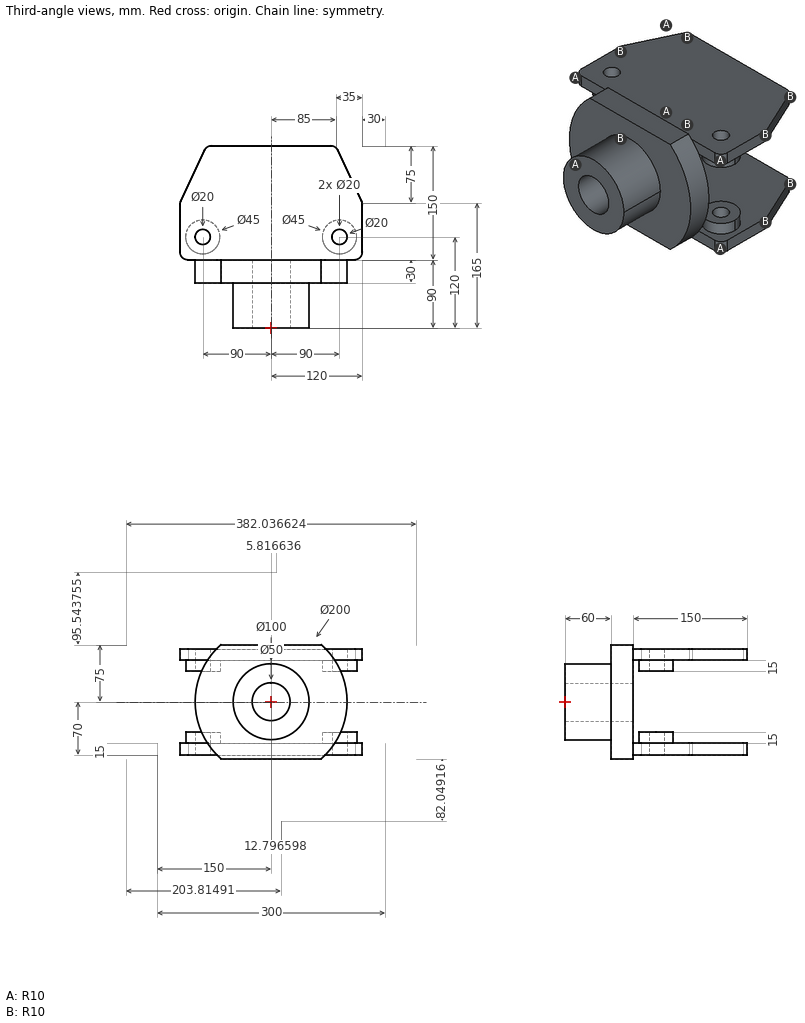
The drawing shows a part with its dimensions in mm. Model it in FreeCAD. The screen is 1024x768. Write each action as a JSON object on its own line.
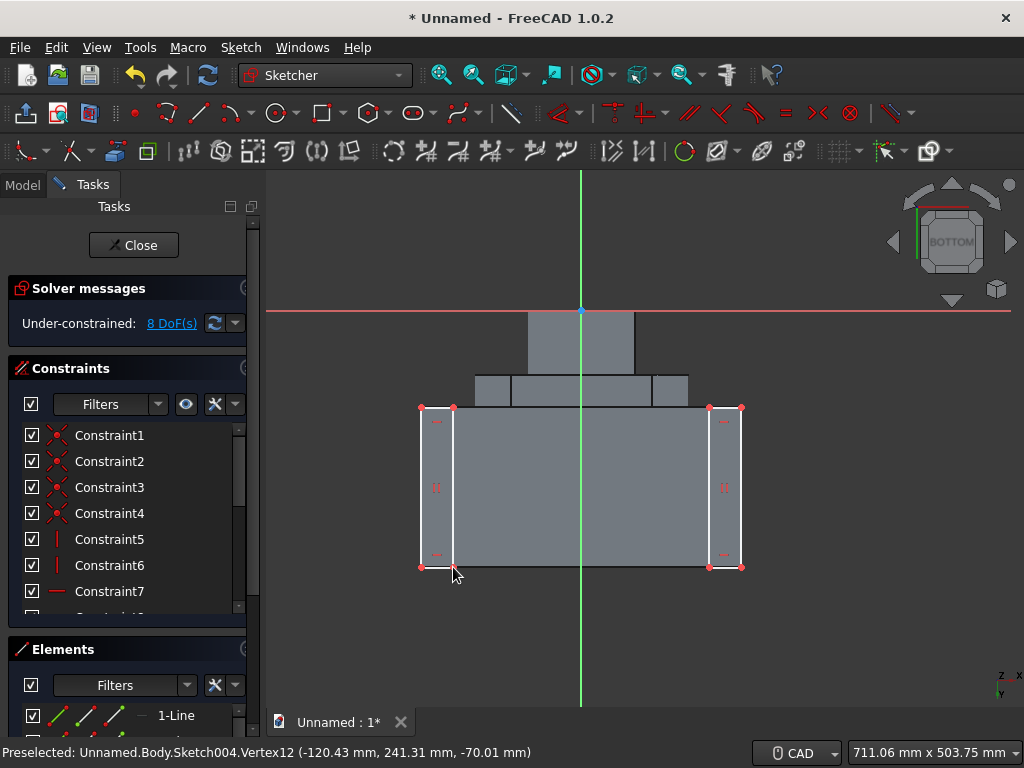
{"action": "left_click", "coordinate": [741, 408]}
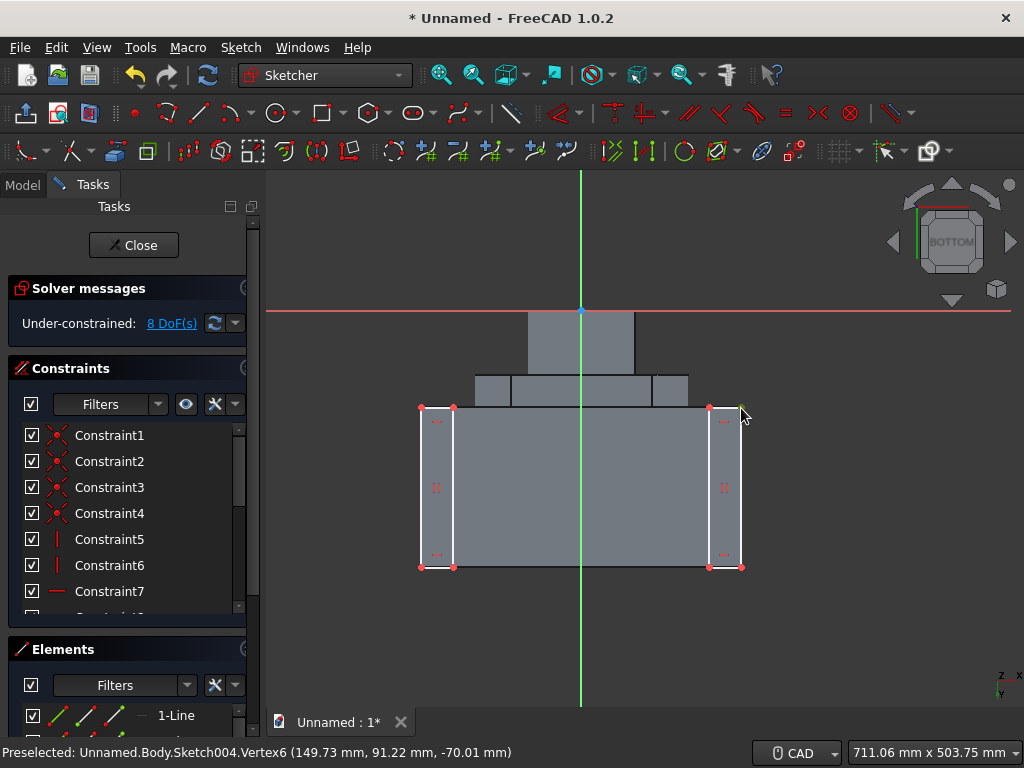
{"action": "left_click", "coordinate": [421, 408]}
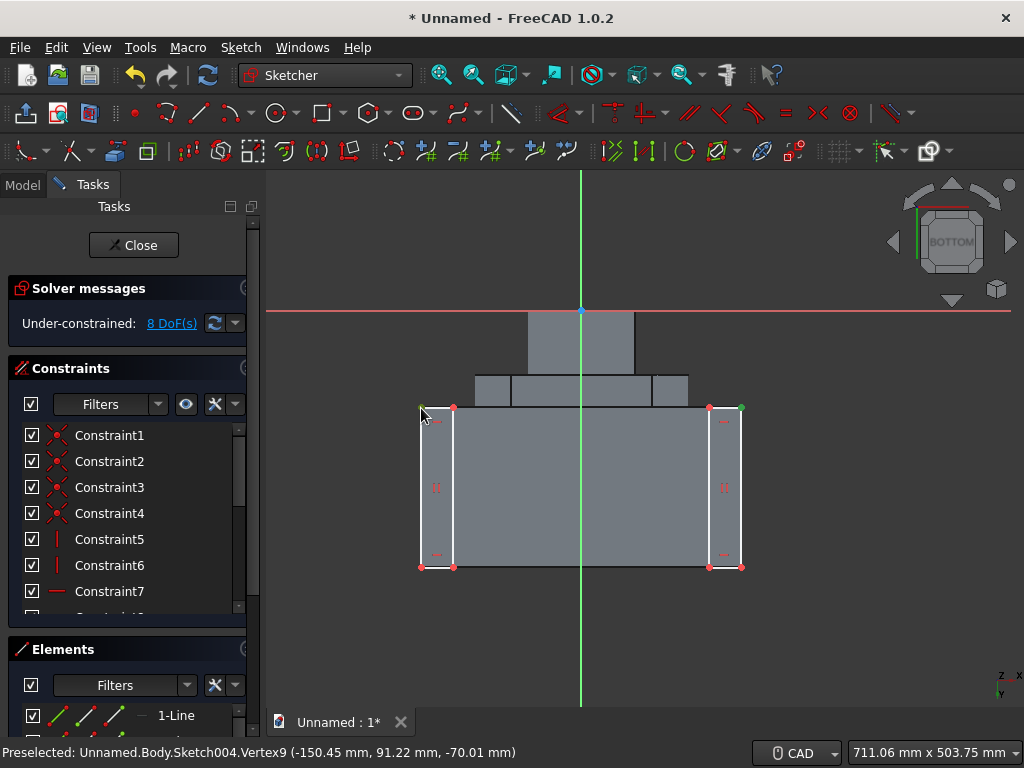
{"action": "left_click", "coordinate": [581, 645]}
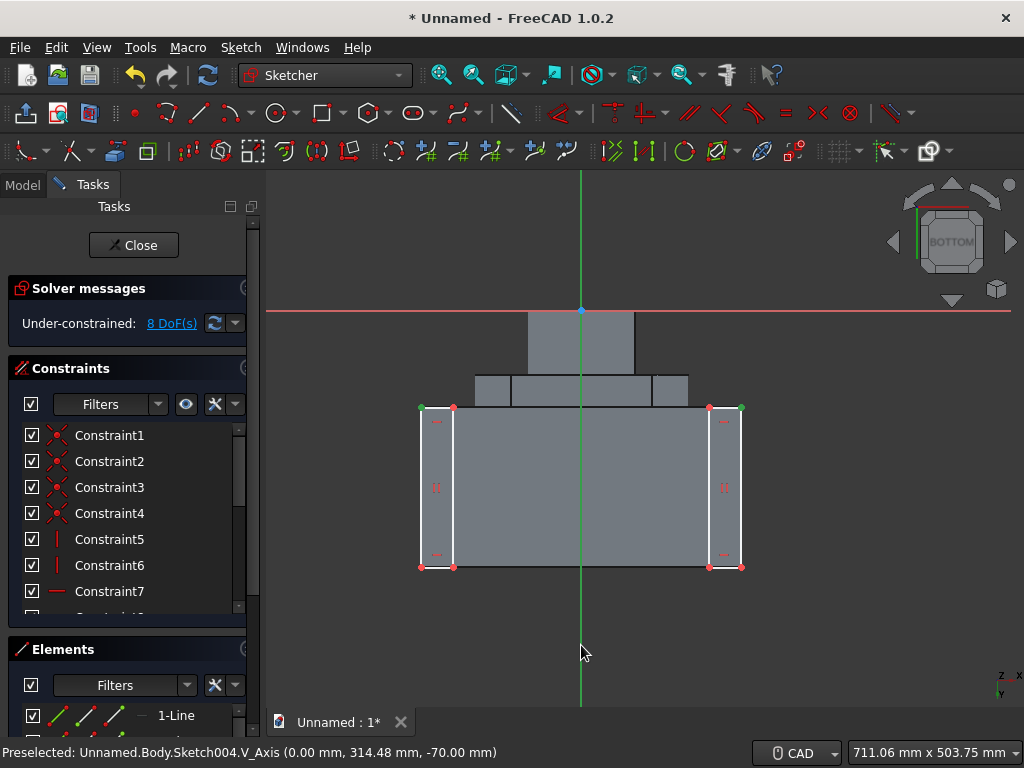
{"action": "left_click", "coordinate": [818, 114]}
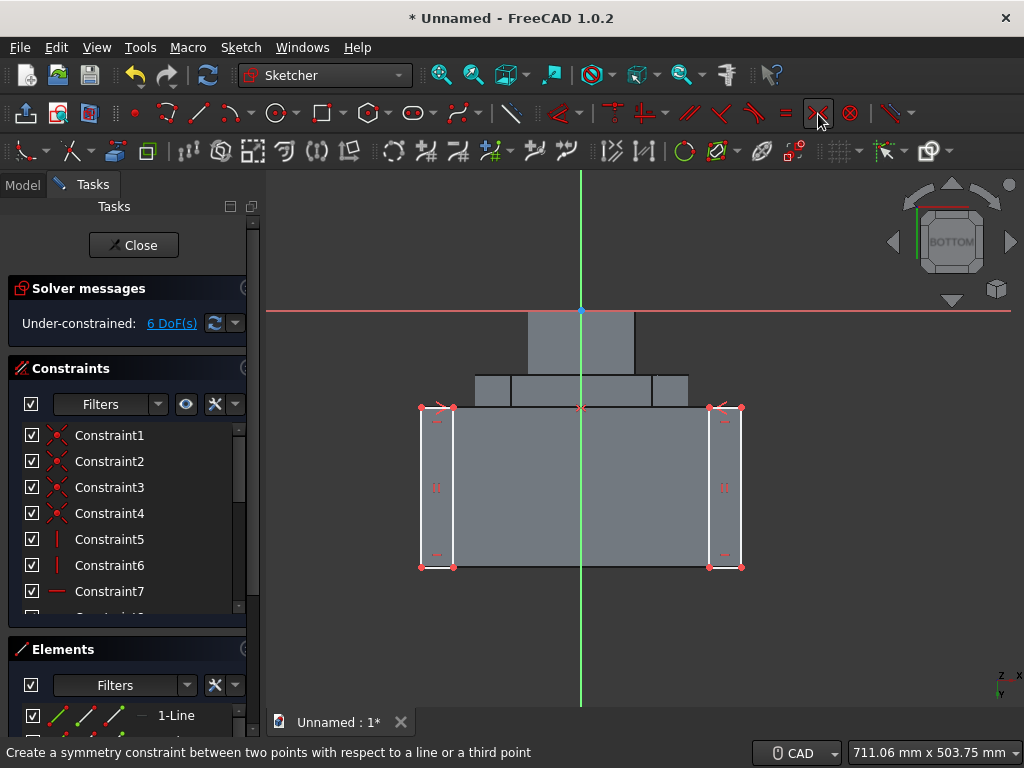
{"action": "left_click", "coordinate": [709, 568]}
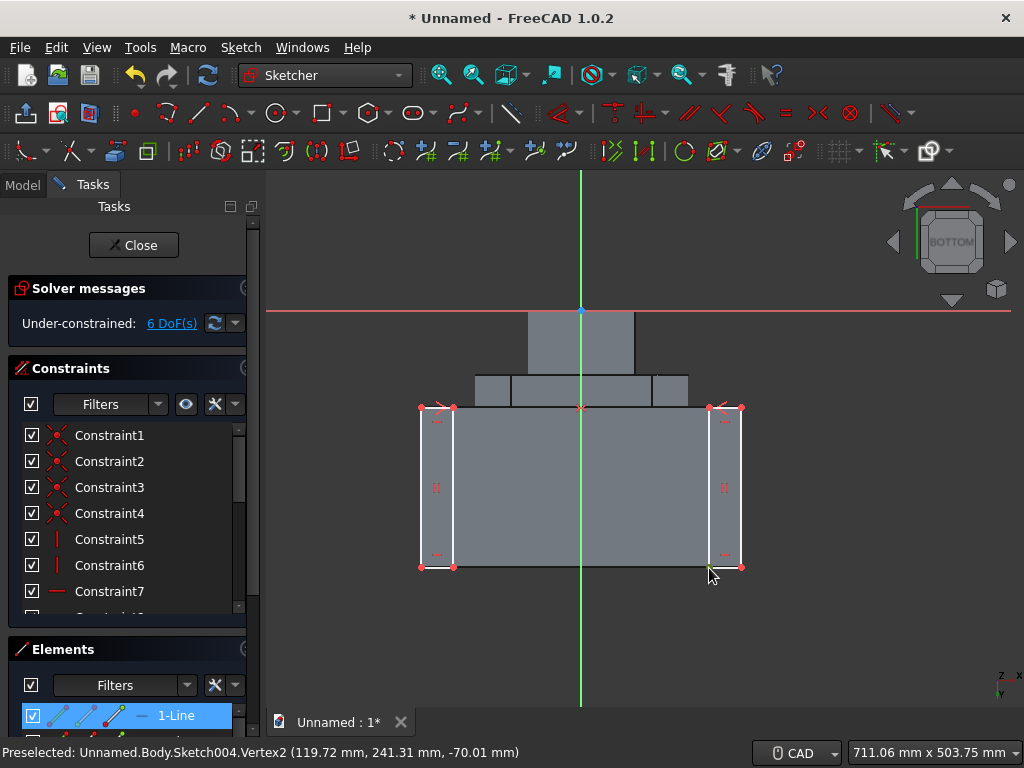
{"action": "left_click", "coordinate": [453, 568]}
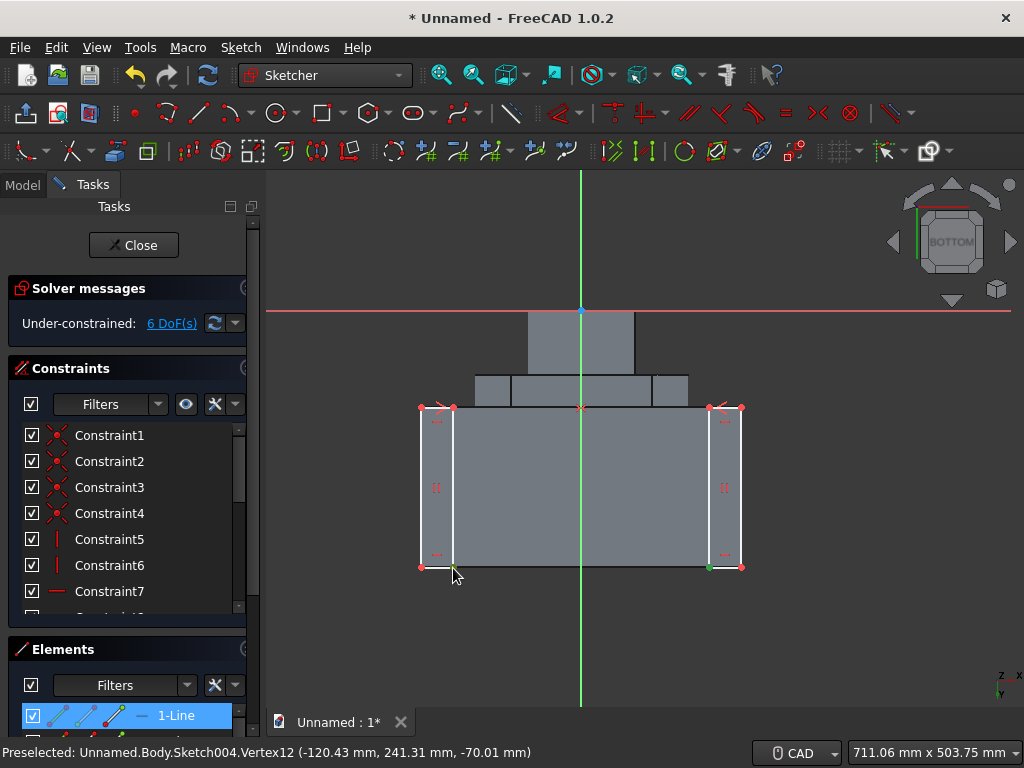
{"action": "left_click", "coordinate": [581, 645]}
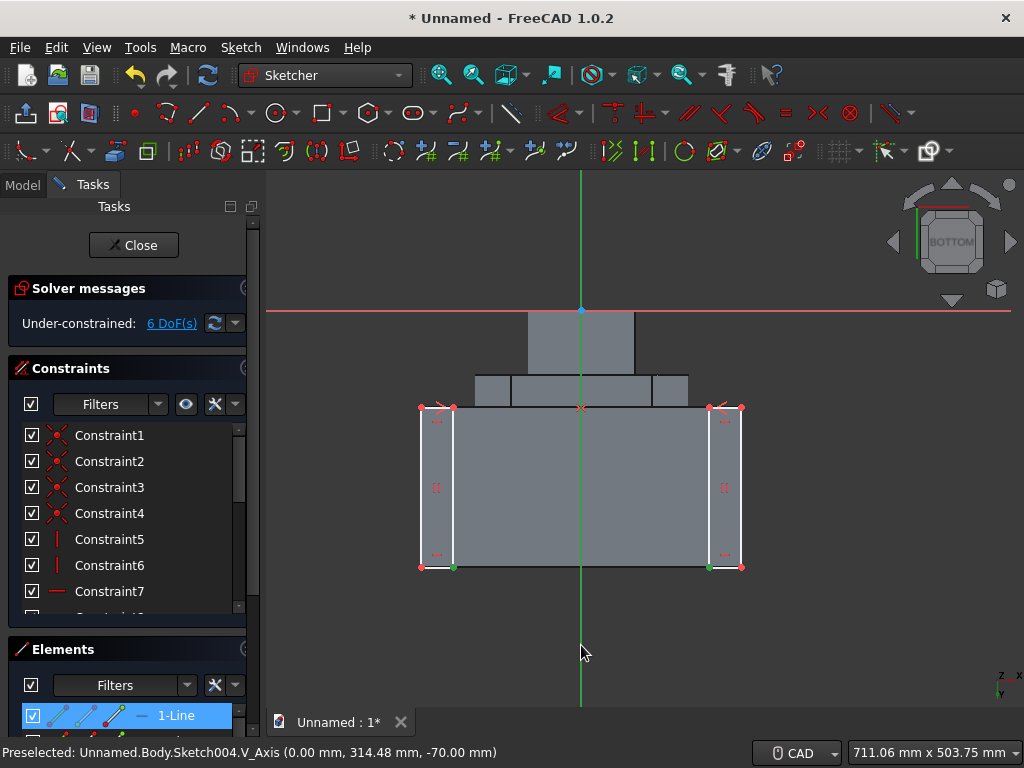
{"action": "left_click", "coordinate": [818, 114]}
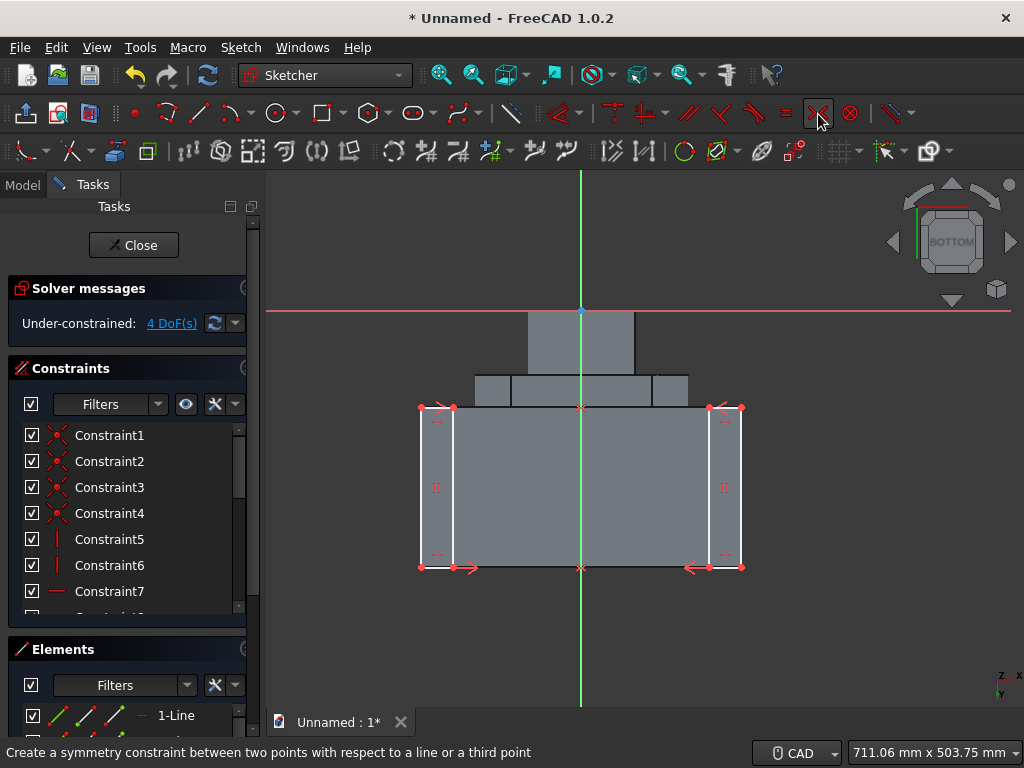
{"action": "key", "text": "d"}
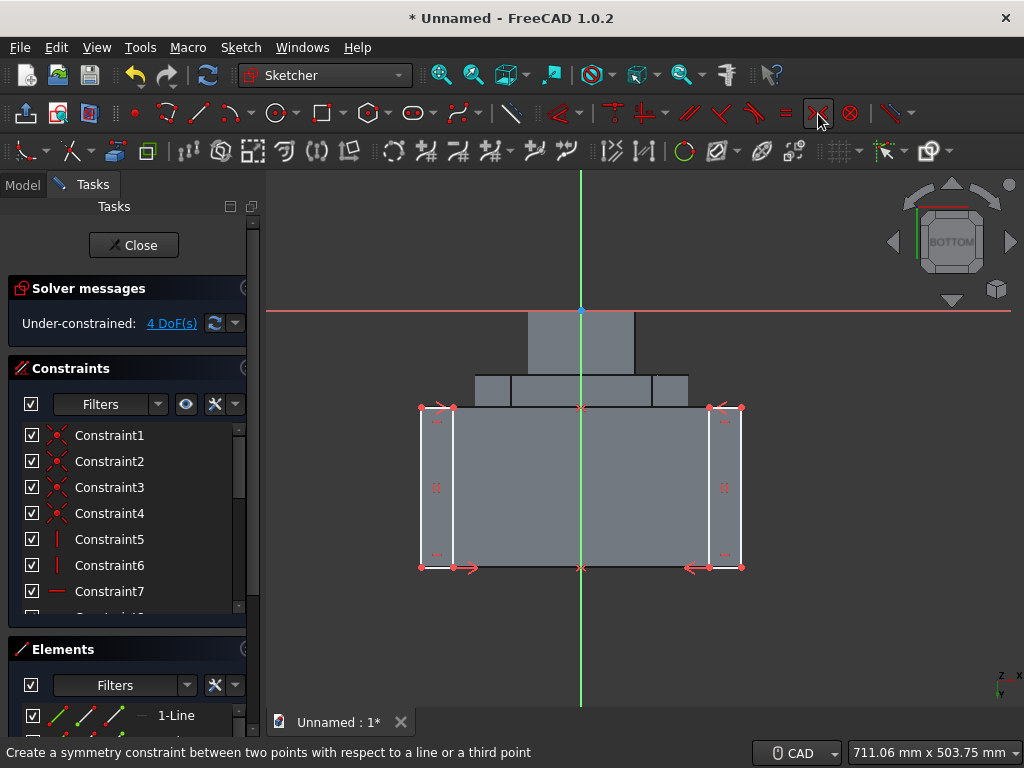
{"action": "scroll", "coordinate": [719, 568], "scroll_direction": "up", "scroll_amount": 2}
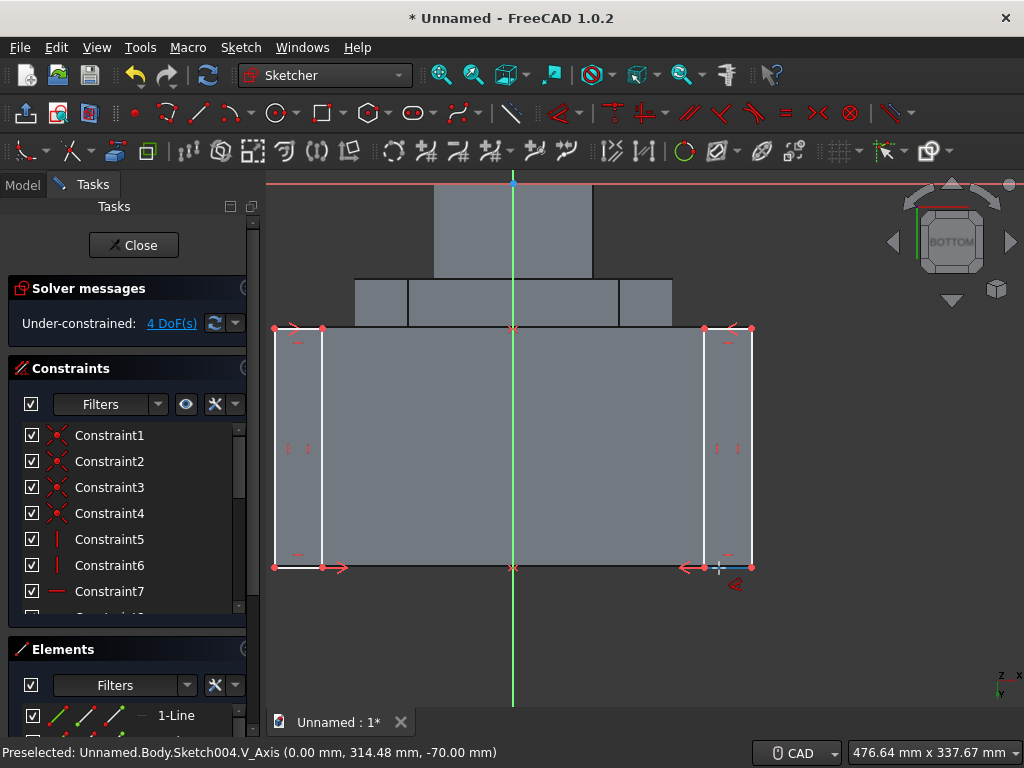
{"action": "left_click", "coordinate": [719, 568]}
{"action": "left_click", "coordinate": [728, 602]}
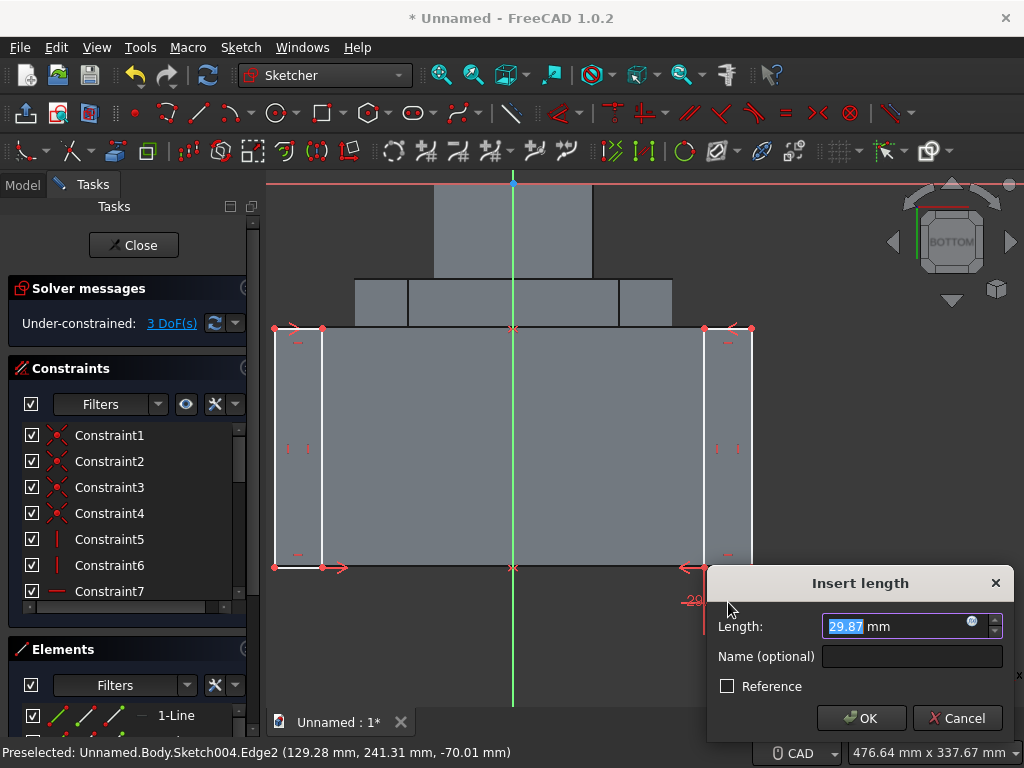
{"action": "type", "text": "30"}
{"action": "key", "text": "Return"}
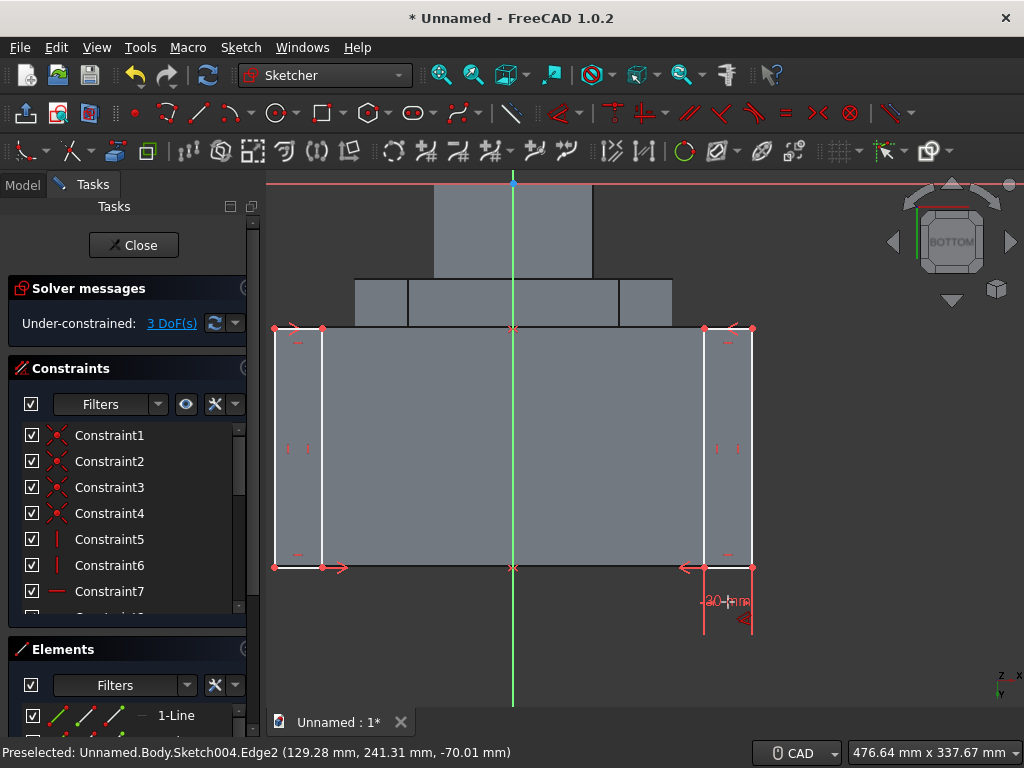
{"action": "left_click", "coordinate": [704, 401]}
{"action": "left_click", "coordinate": [738, 448]}